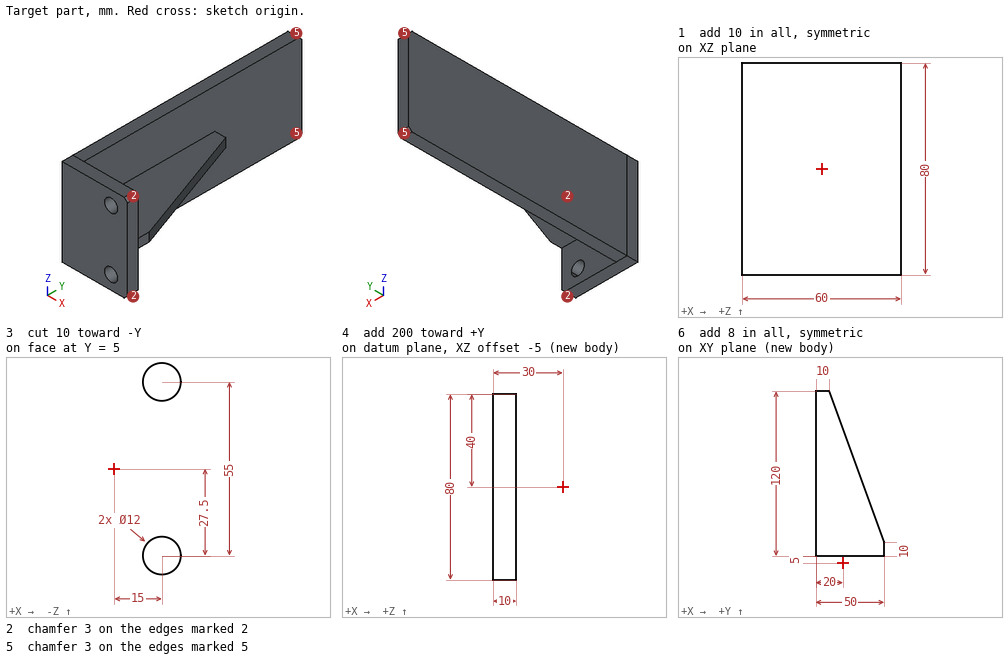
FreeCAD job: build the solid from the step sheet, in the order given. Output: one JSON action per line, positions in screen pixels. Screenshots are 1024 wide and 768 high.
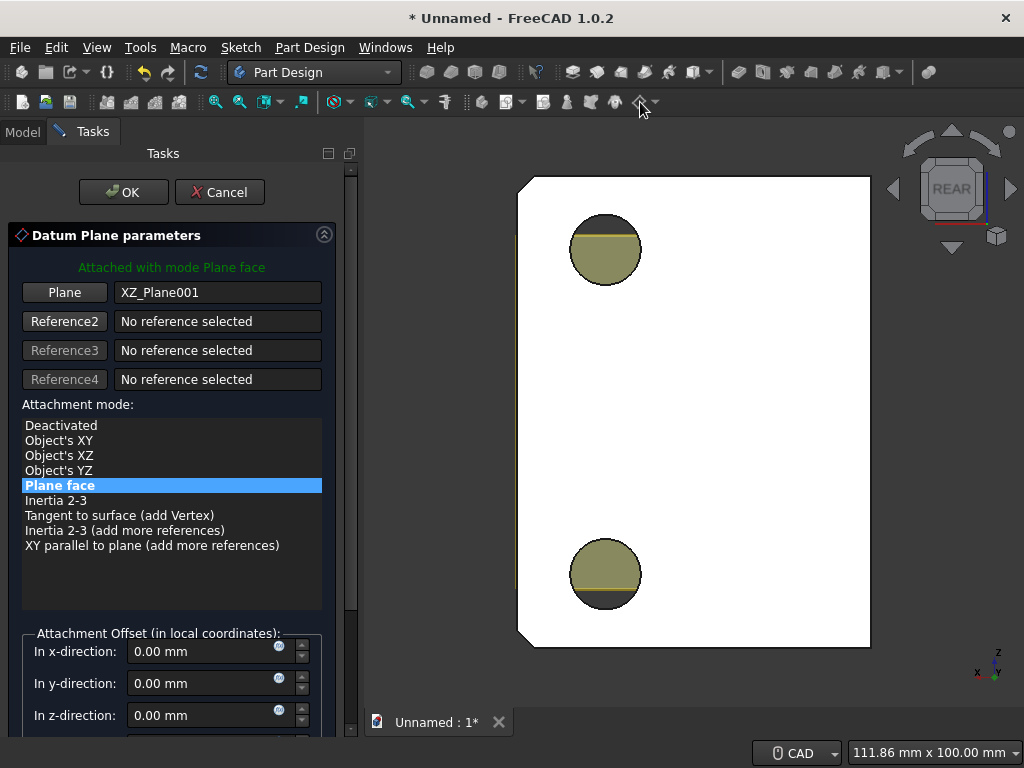
{"action": "triple_click", "coordinate": [210, 715]}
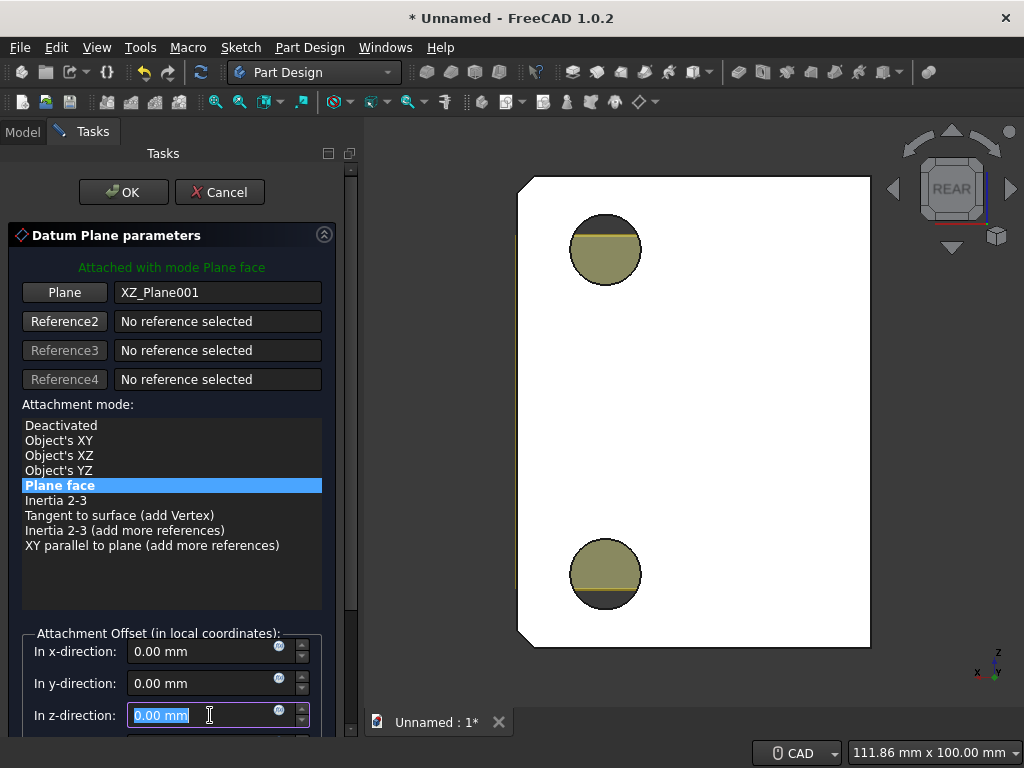
{"action": "type", "text": "-5"}
{"action": "key", "text": "Tab"}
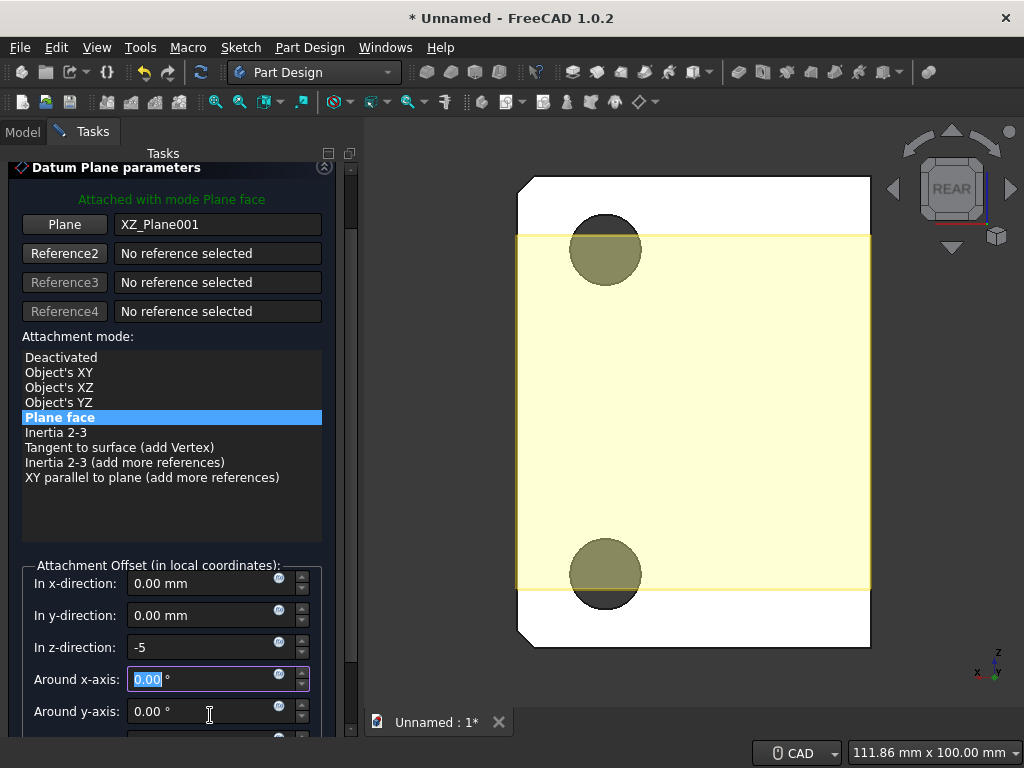
{"action": "scroll", "coordinate": [351, 450], "scroll_direction": "up", "scroll_amount": 2}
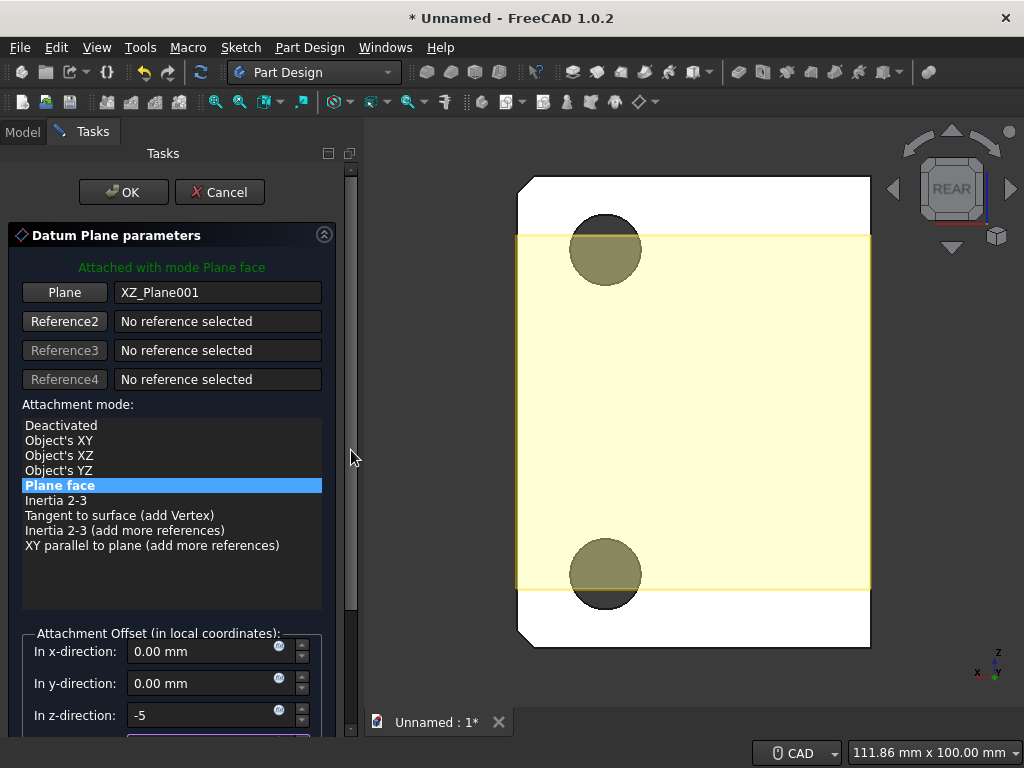
{"action": "left_click", "coordinate": [124, 192]}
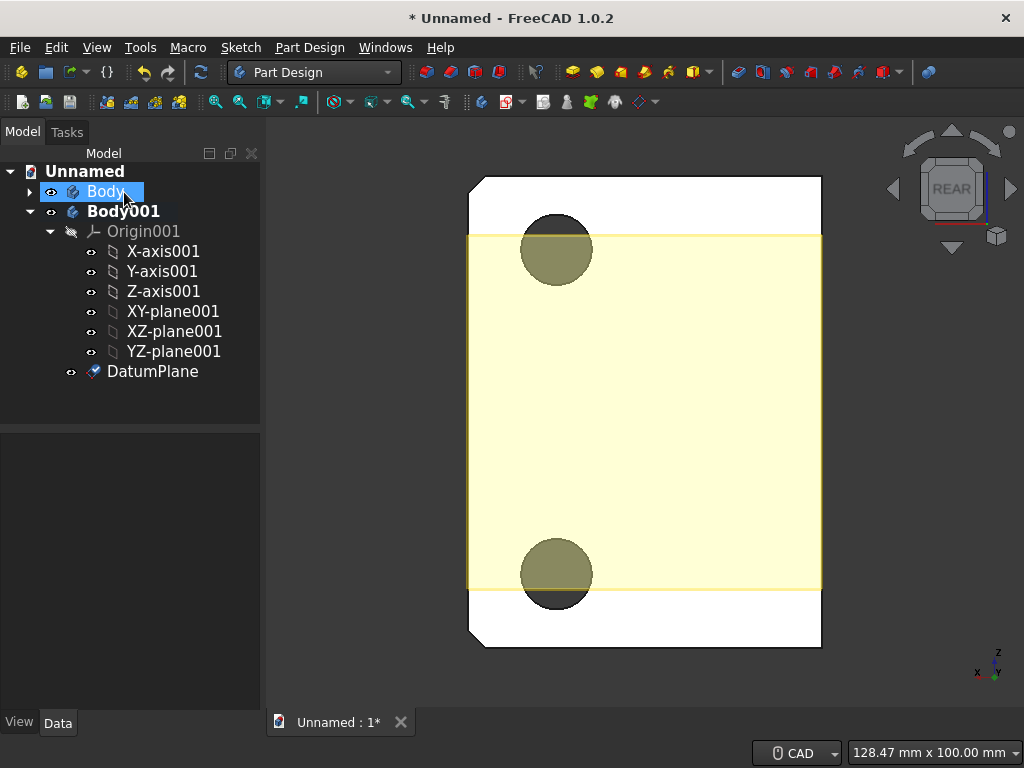
{"action": "left_click", "coordinate": [116, 372]}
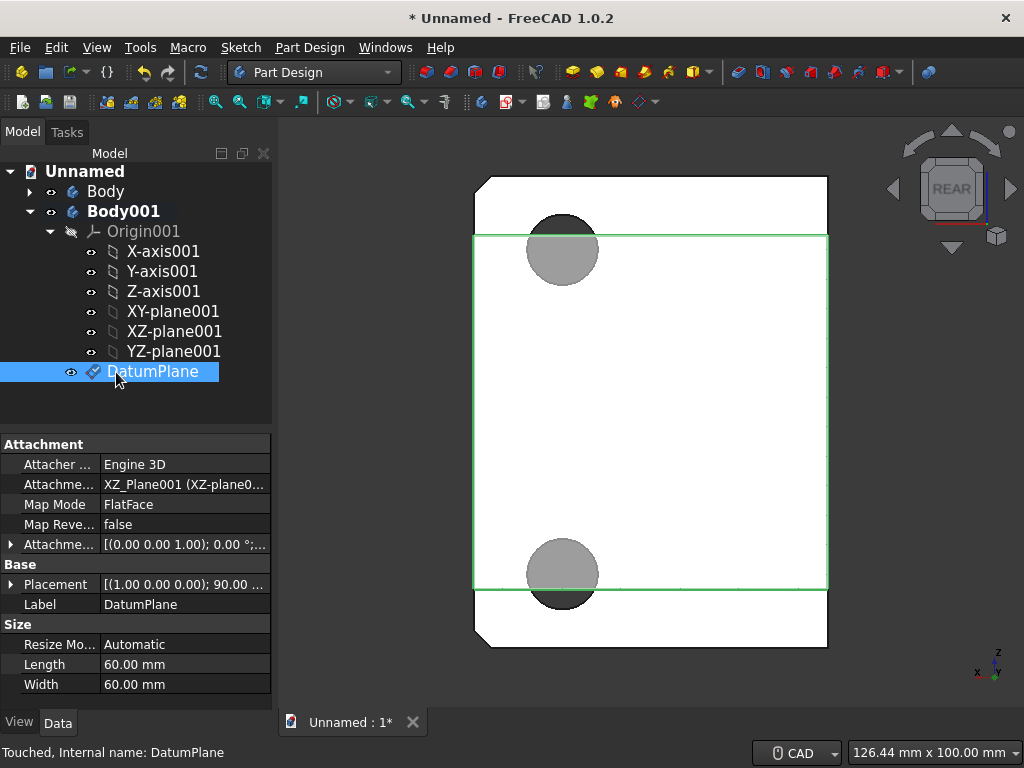
{"action": "left_click", "coordinate": [506, 102]}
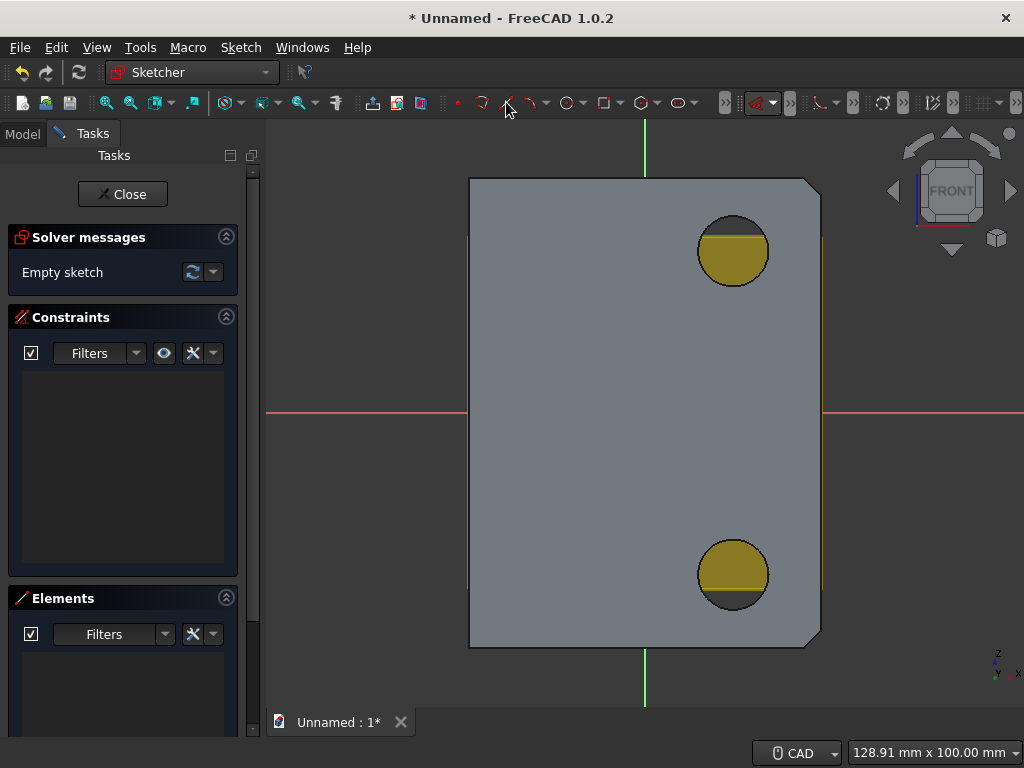
{"action": "left_click", "coordinate": [604, 104]}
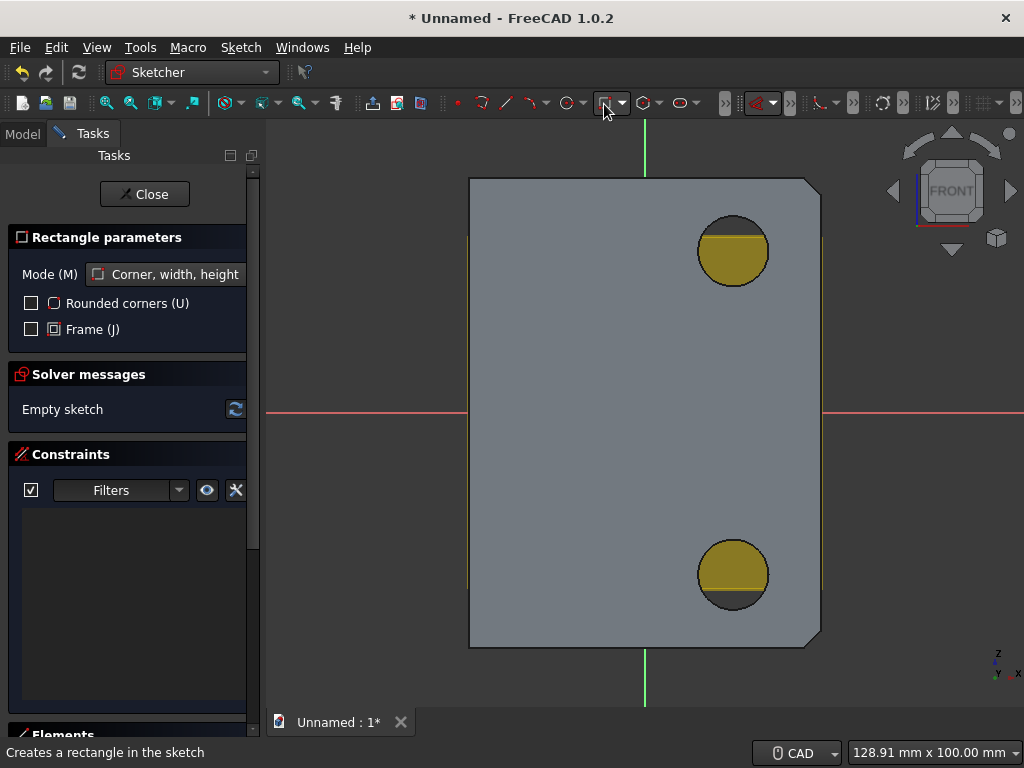
{"action": "left_click", "coordinate": [469, 178]}
{"action": "mouse_move", "coordinate": [527, 648]}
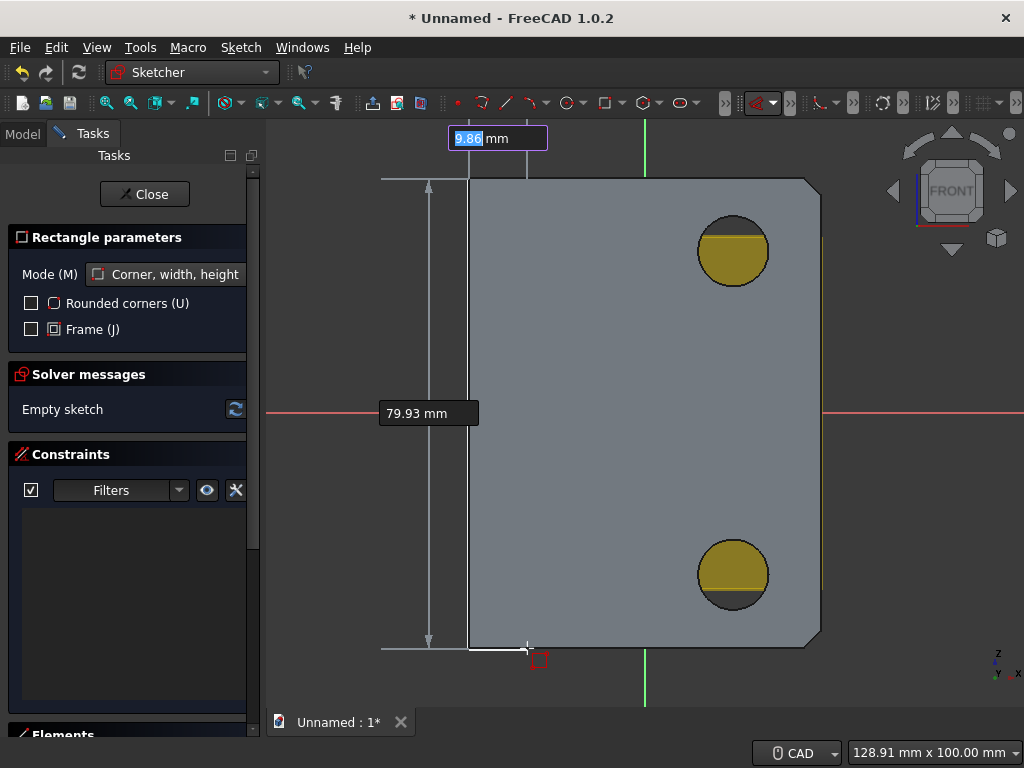
{"action": "type", "text": "10"}
{"action": "key", "text": "Tab"}
{"action": "type", "text": "80"}
{"action": "key", "text": "Return"}
{"action": "key", "text": "Escape"}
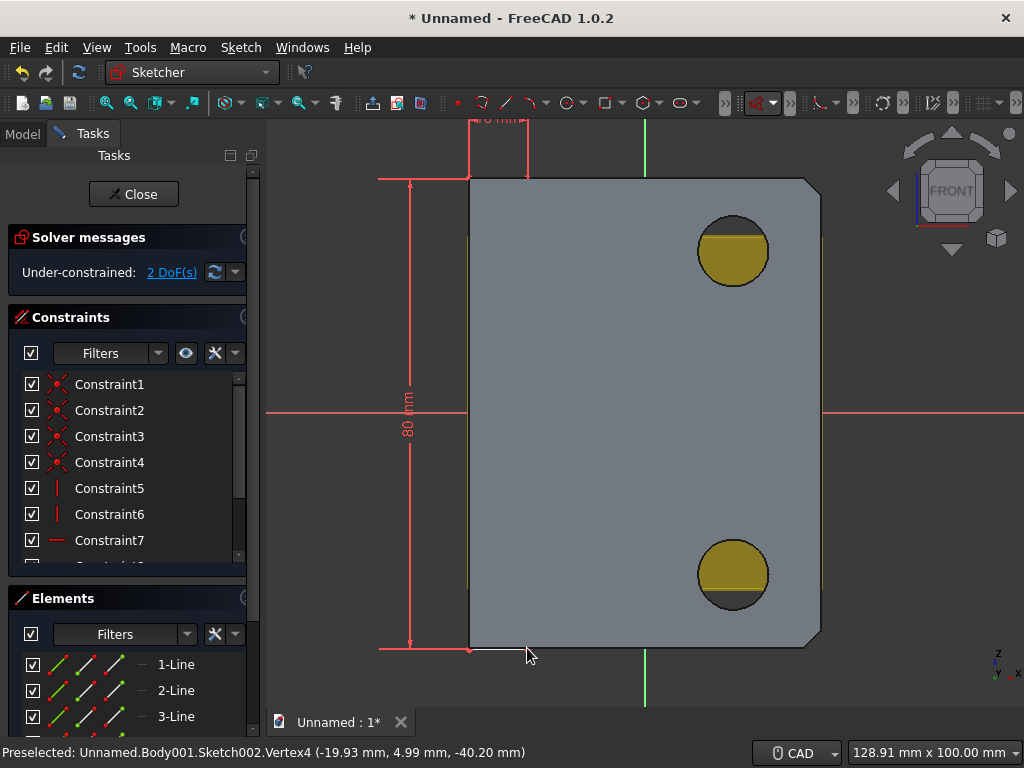
{"action": "left_click", "coordinate": [469, 179]}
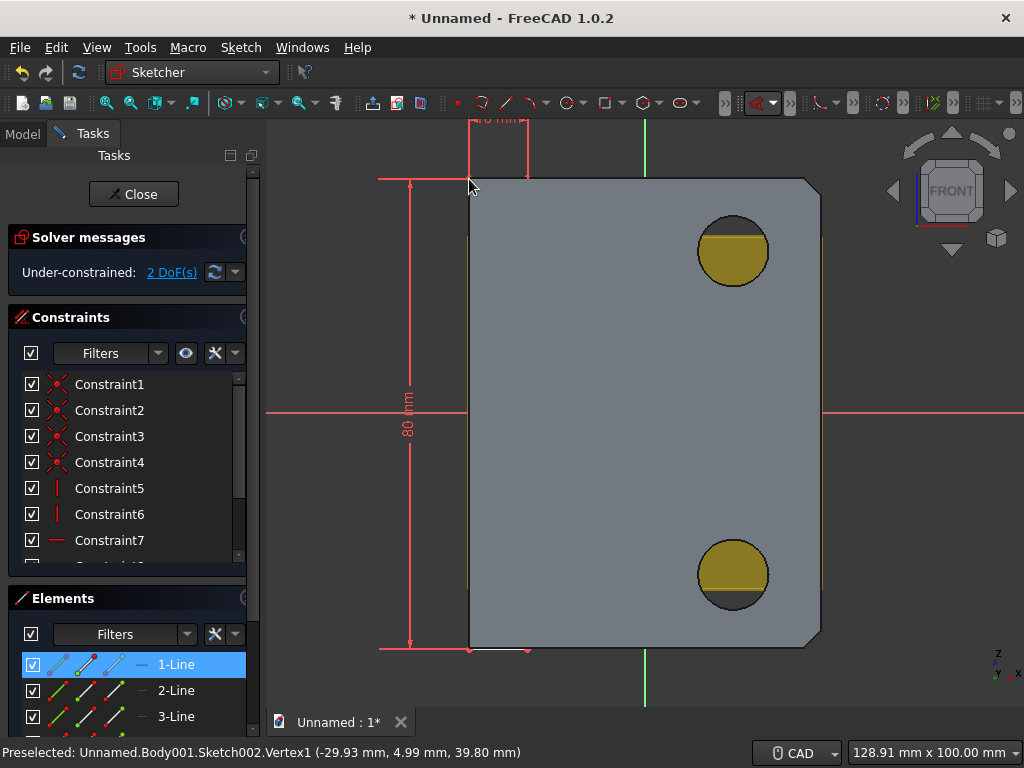
{"action": "key", "text": "l"}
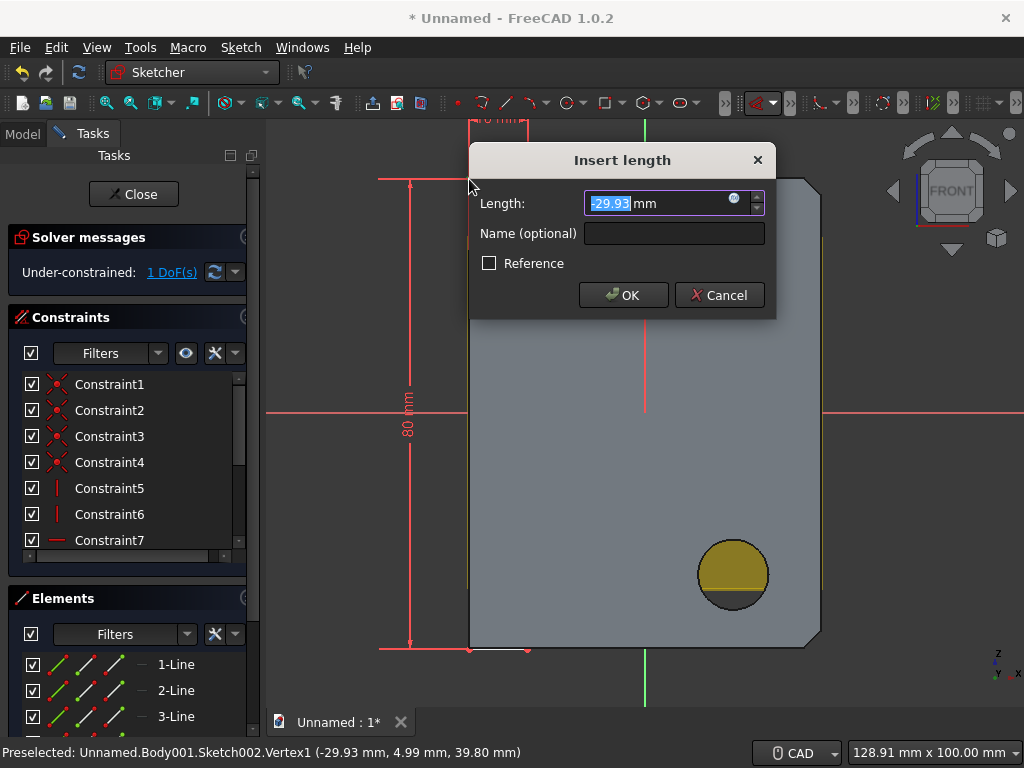
{"action": "type", "text": "-30"}
{"action": "key", "text": "Return"}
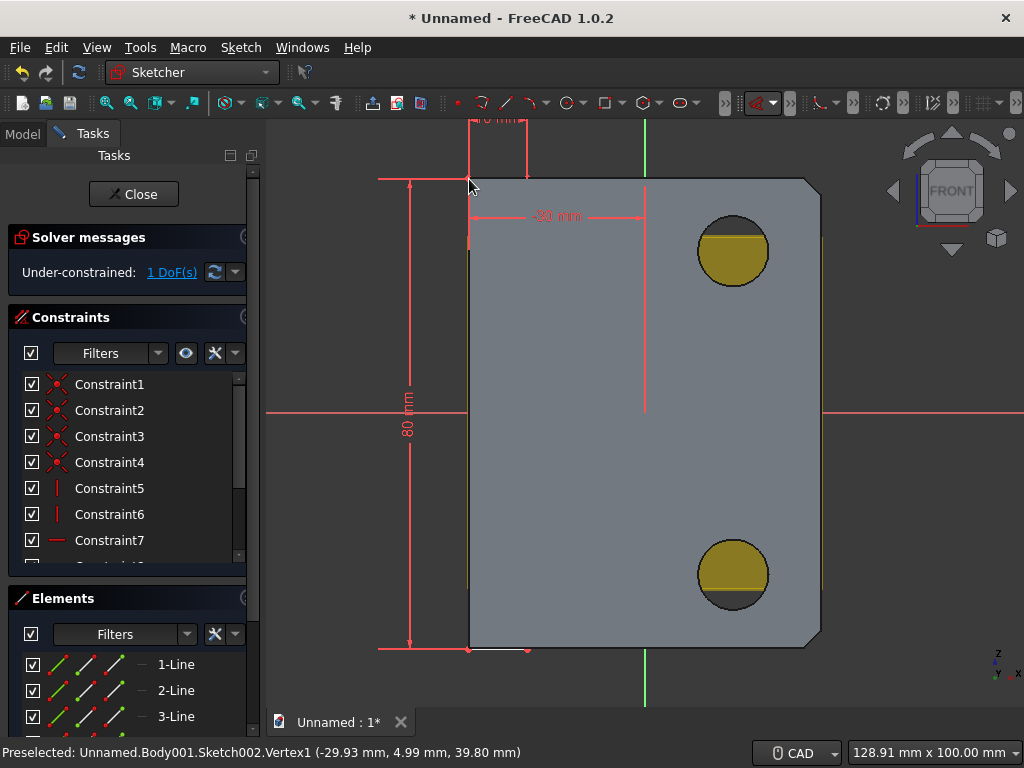
{"action": "left_click", "coordinate": [469, 179]}